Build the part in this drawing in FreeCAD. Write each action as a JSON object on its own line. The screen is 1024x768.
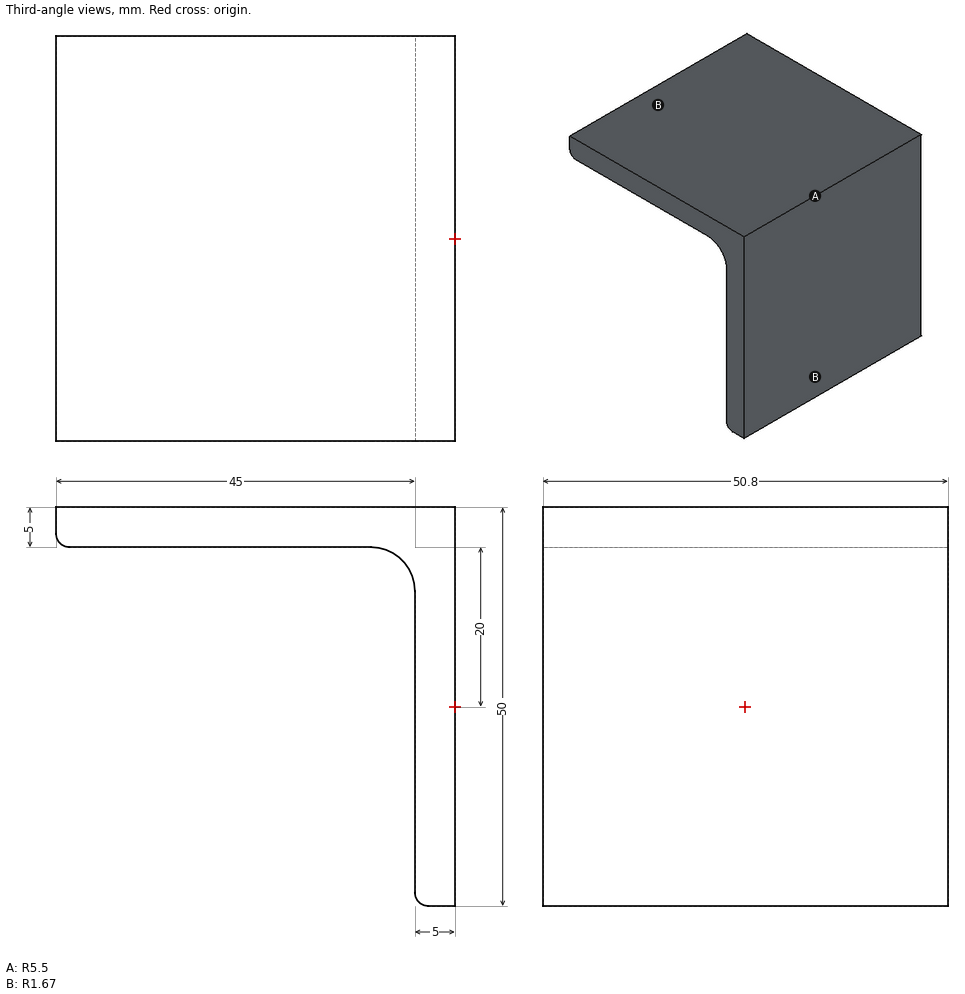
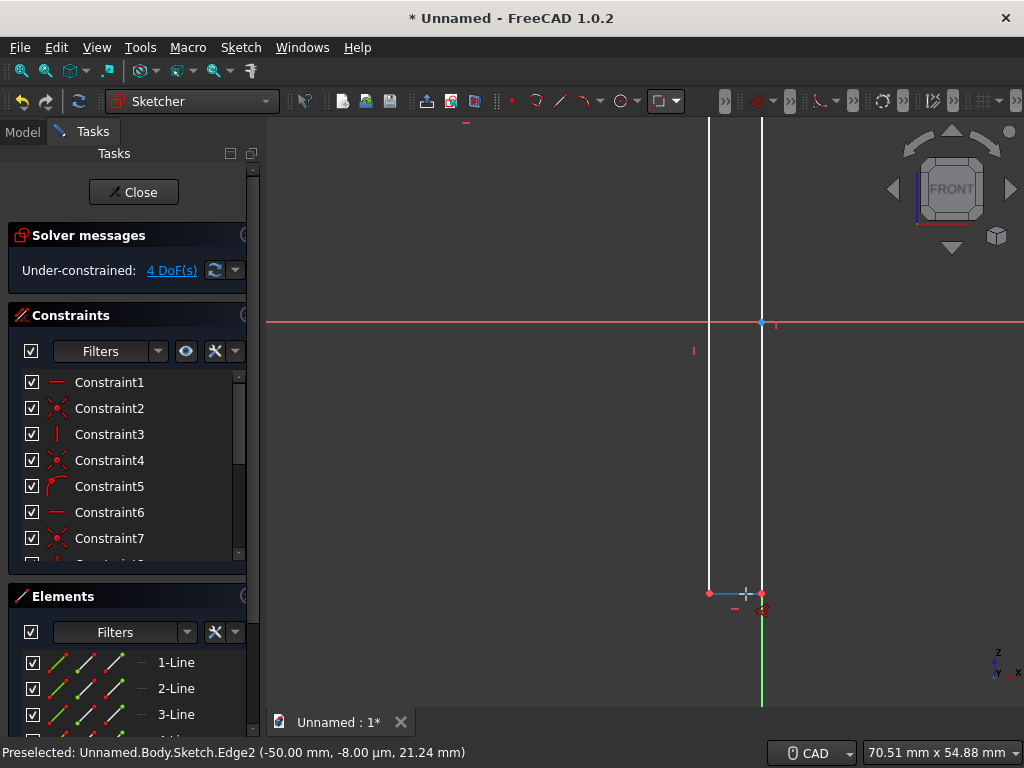
{"action": "left_click", "coordinate": [746, 594]}
{"action": "left_click", "coordinate": [735, 628]}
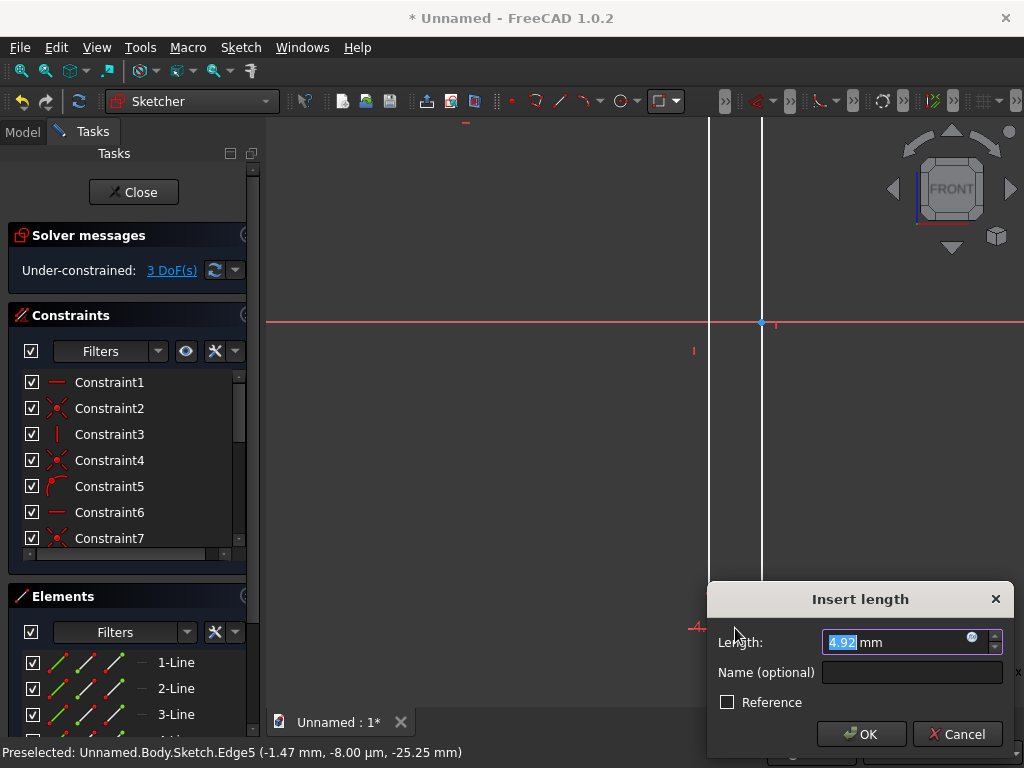
{"action": "type", "text": "5"}
{"action": "key", "text": "Return"}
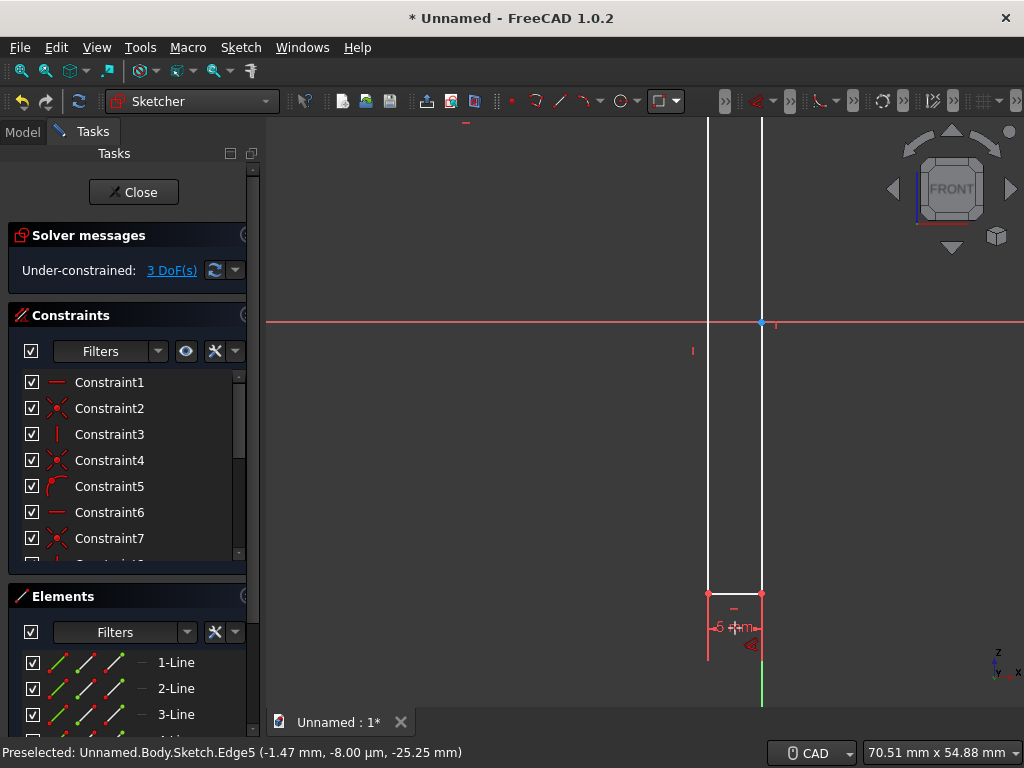
{"action": "scroll", "coordinate": [746, 595], "scroll_direction": "down", "scroll_amount": 2}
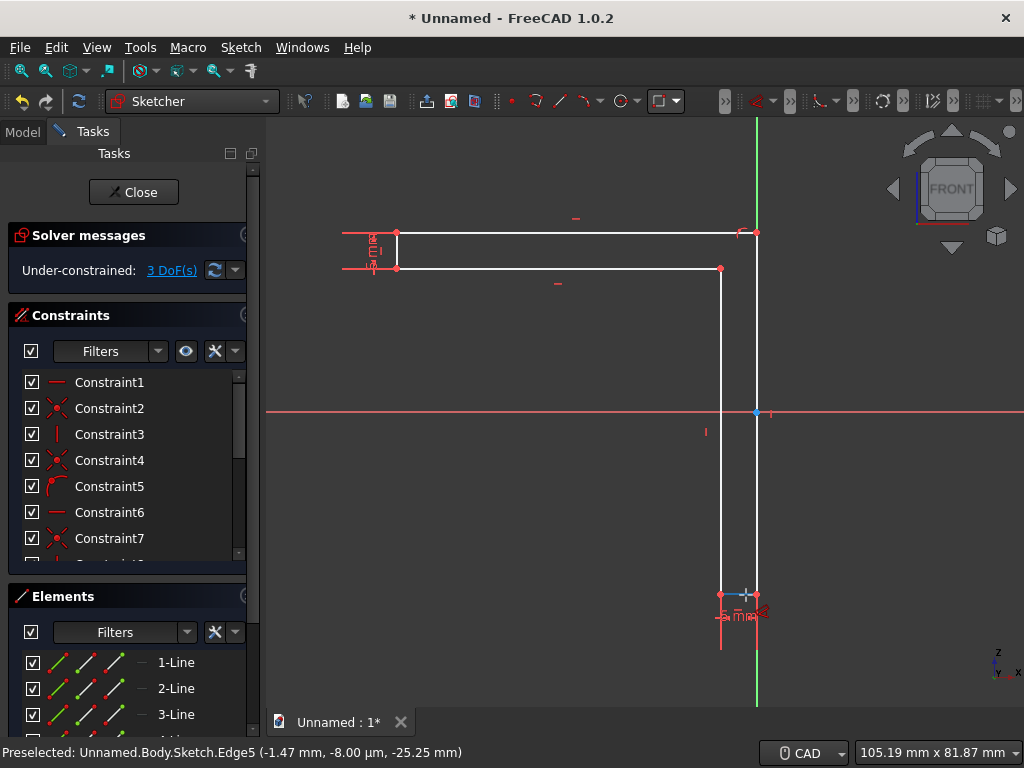
{"action": "left_click", "coordinate": [624, 269]}
{"action": "left_click", "coordinate": [559, 303]}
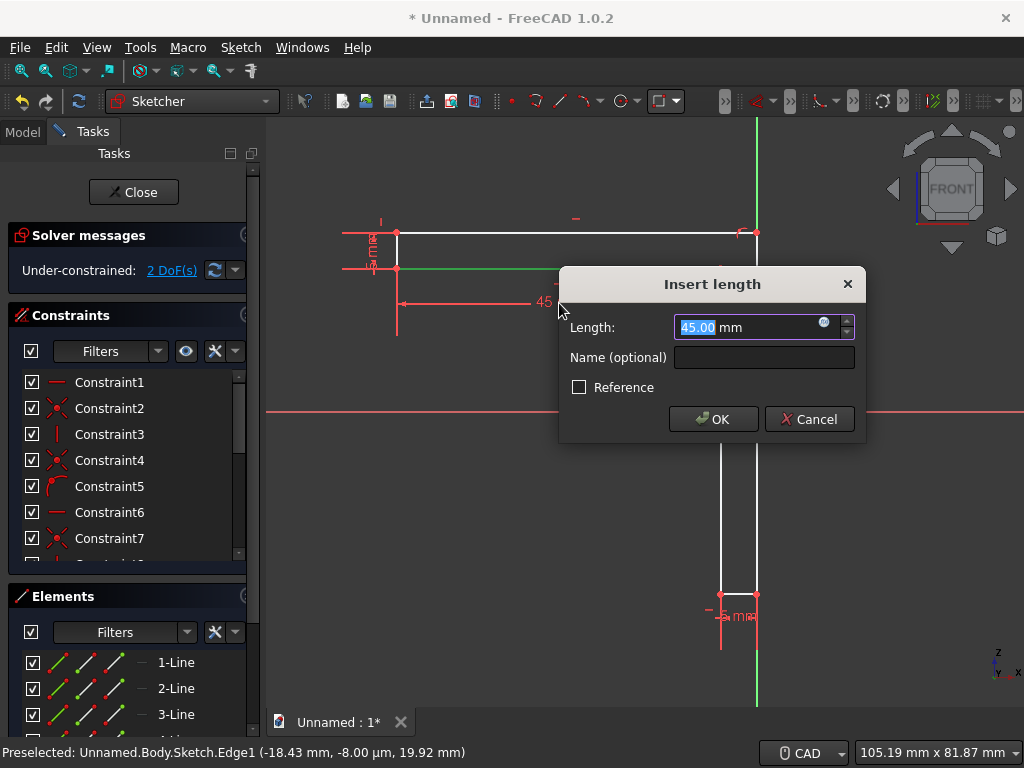
{"action": "type", "text": "45"}
{"action": "key", "text": "Return"}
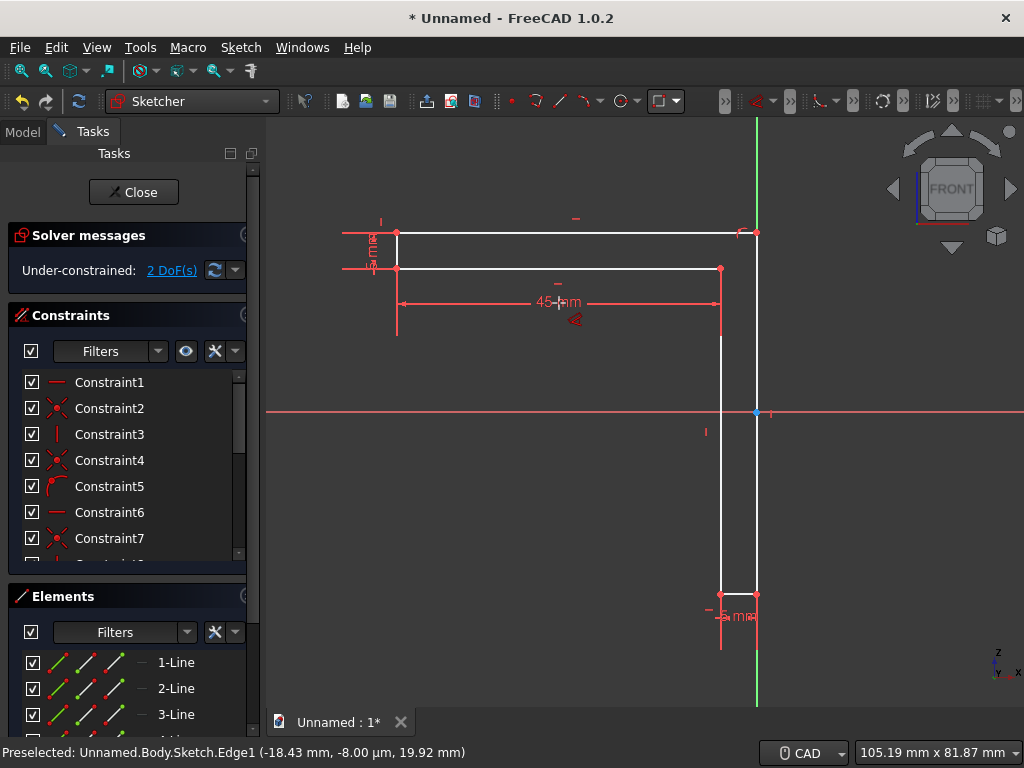
{"action": "left_click", "coordinate": [757, 341]}
{"action": "left_click", "coordinate": [791, 330]}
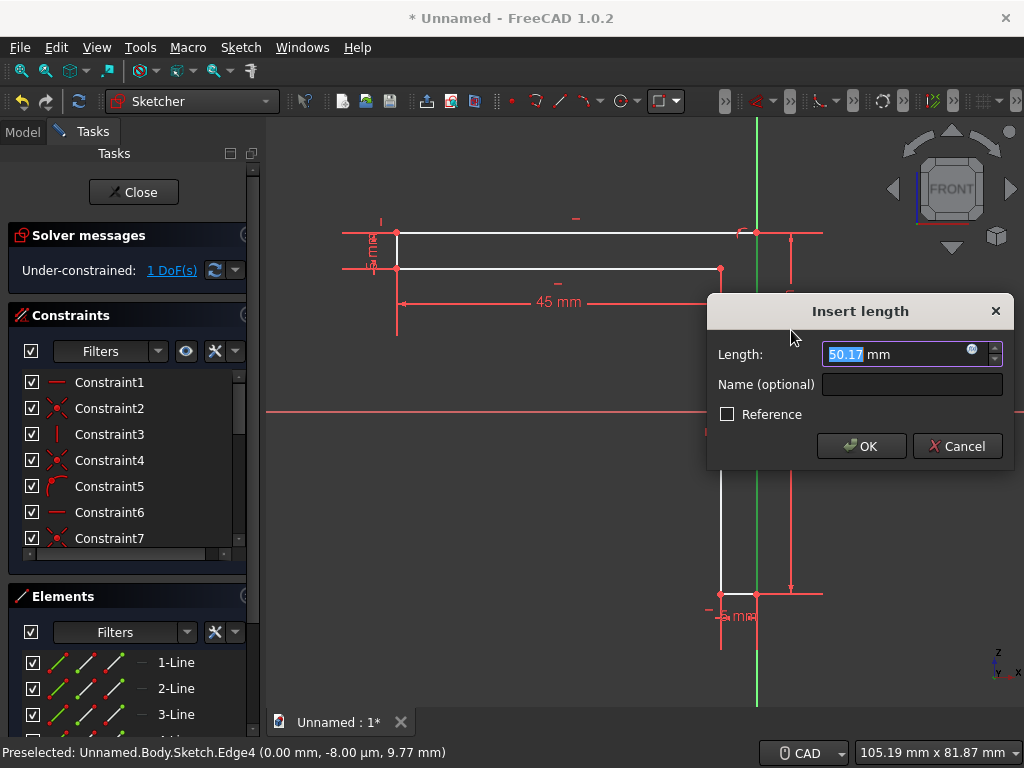
{"action": "type", "text": "50"}
{"action": "key", "text": "Return"}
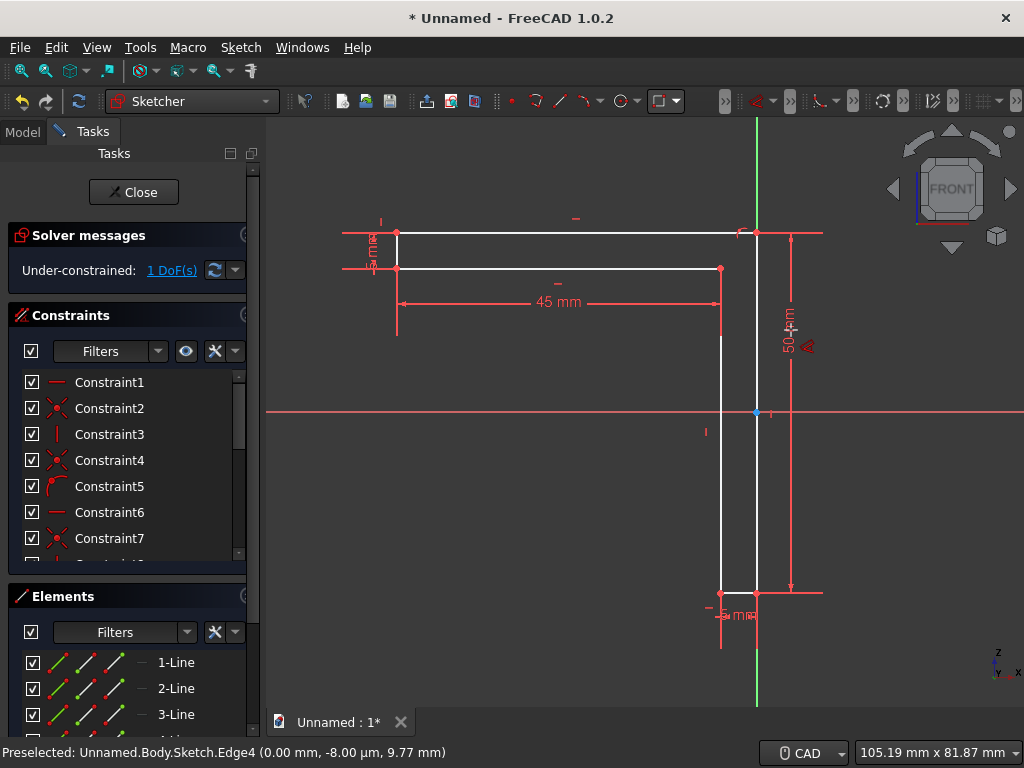
{"action": "left_click", "coordinate": [721, 269]}
{"action": "left_click", "coordinate": [791, 308]}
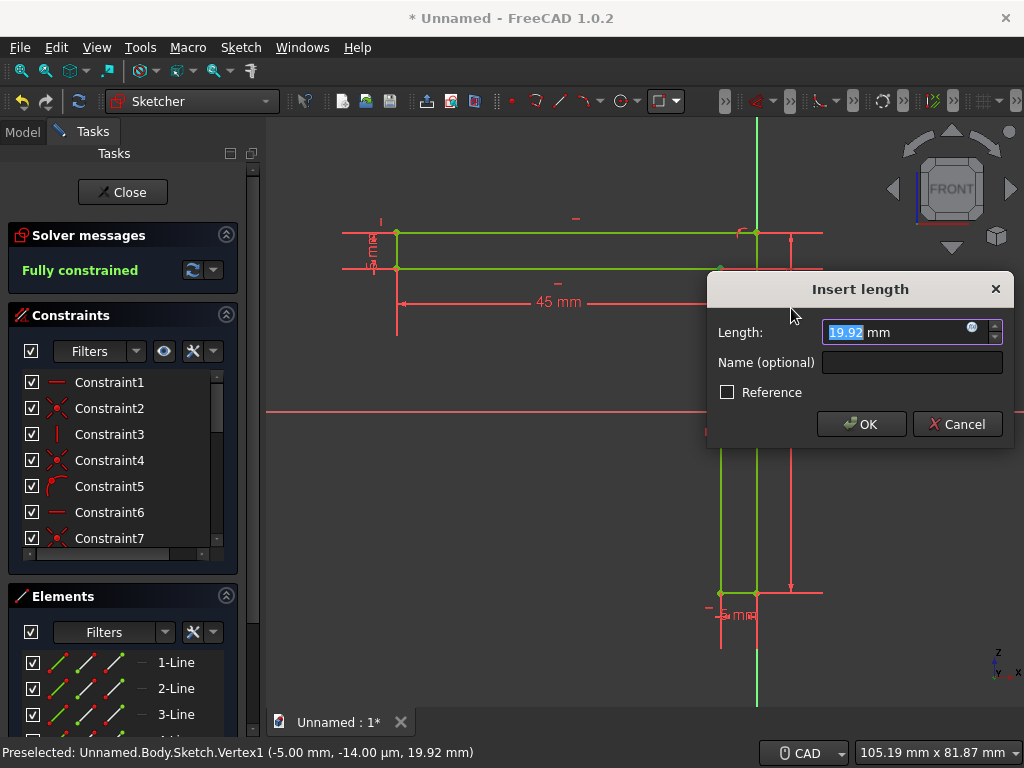
{"action": "type", "text": "20"}
{"action": "key", "text": "Return"}
{"action": "key", "text": "Escape"}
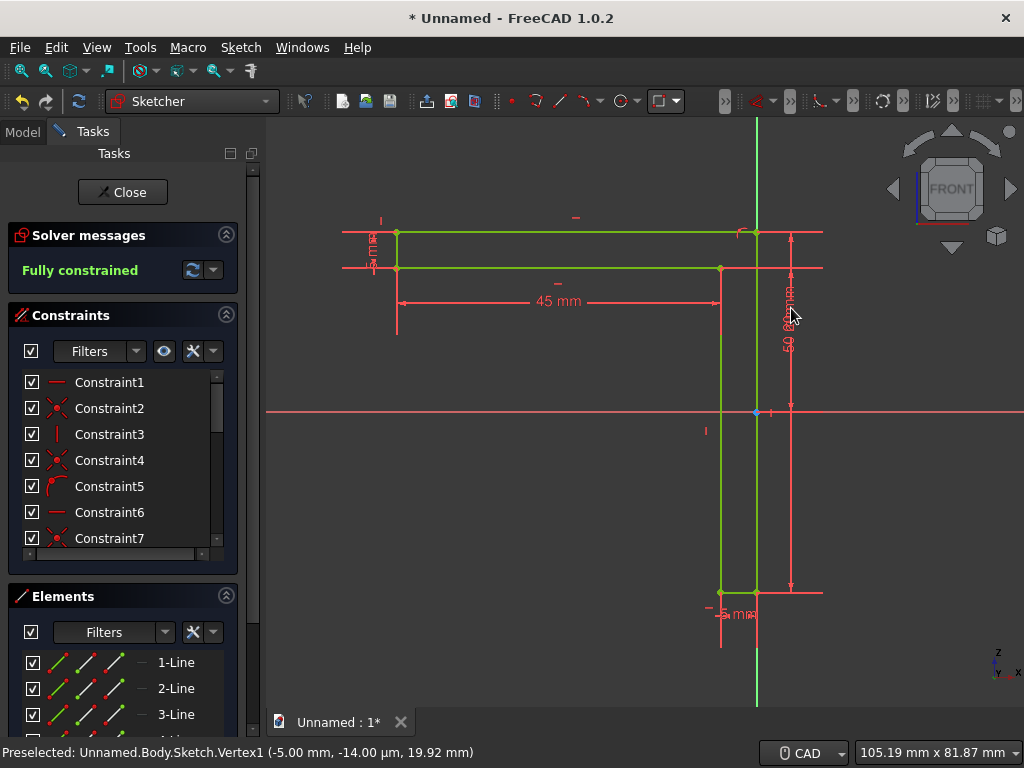
{"action": "left_click", "coordinate": [123, 192]}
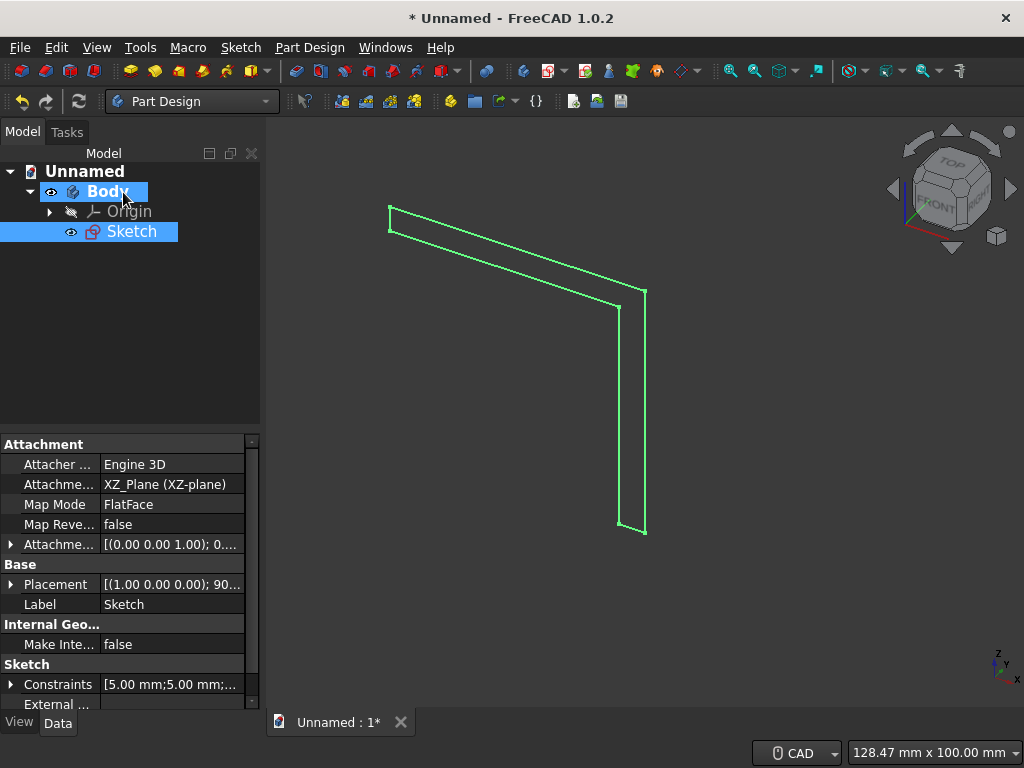
{"action": "left_click", "coordinate": [132, 72]}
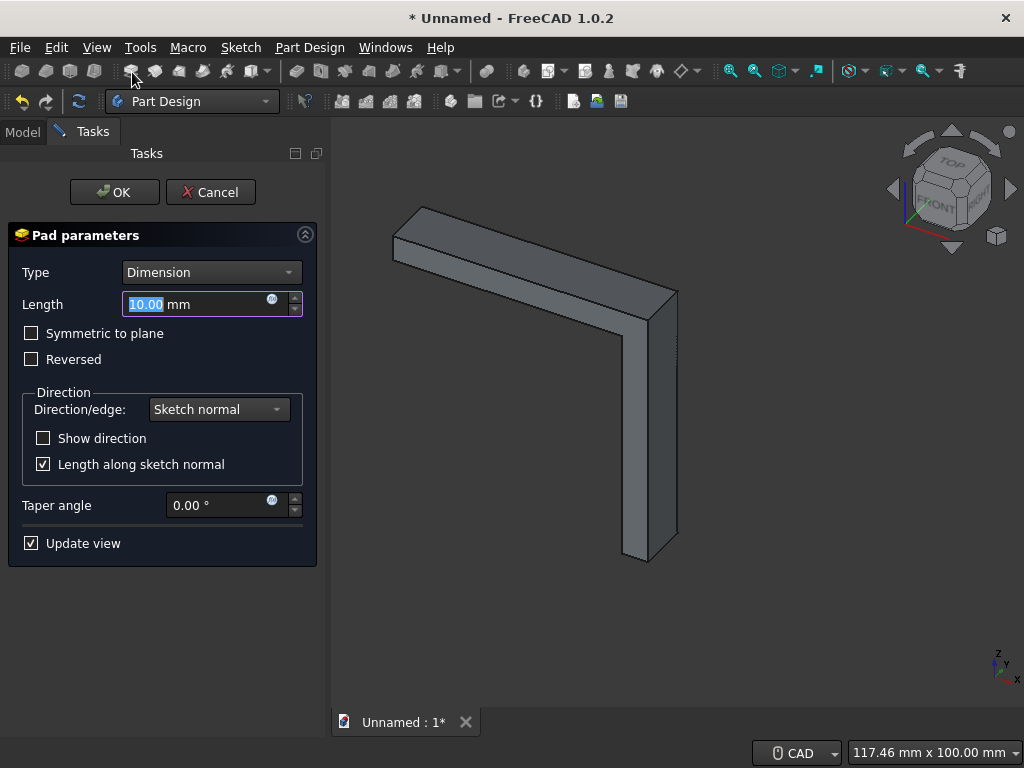
{"action": "type", "text": "50.8"}
{"action": "key", "text": "Tab"}